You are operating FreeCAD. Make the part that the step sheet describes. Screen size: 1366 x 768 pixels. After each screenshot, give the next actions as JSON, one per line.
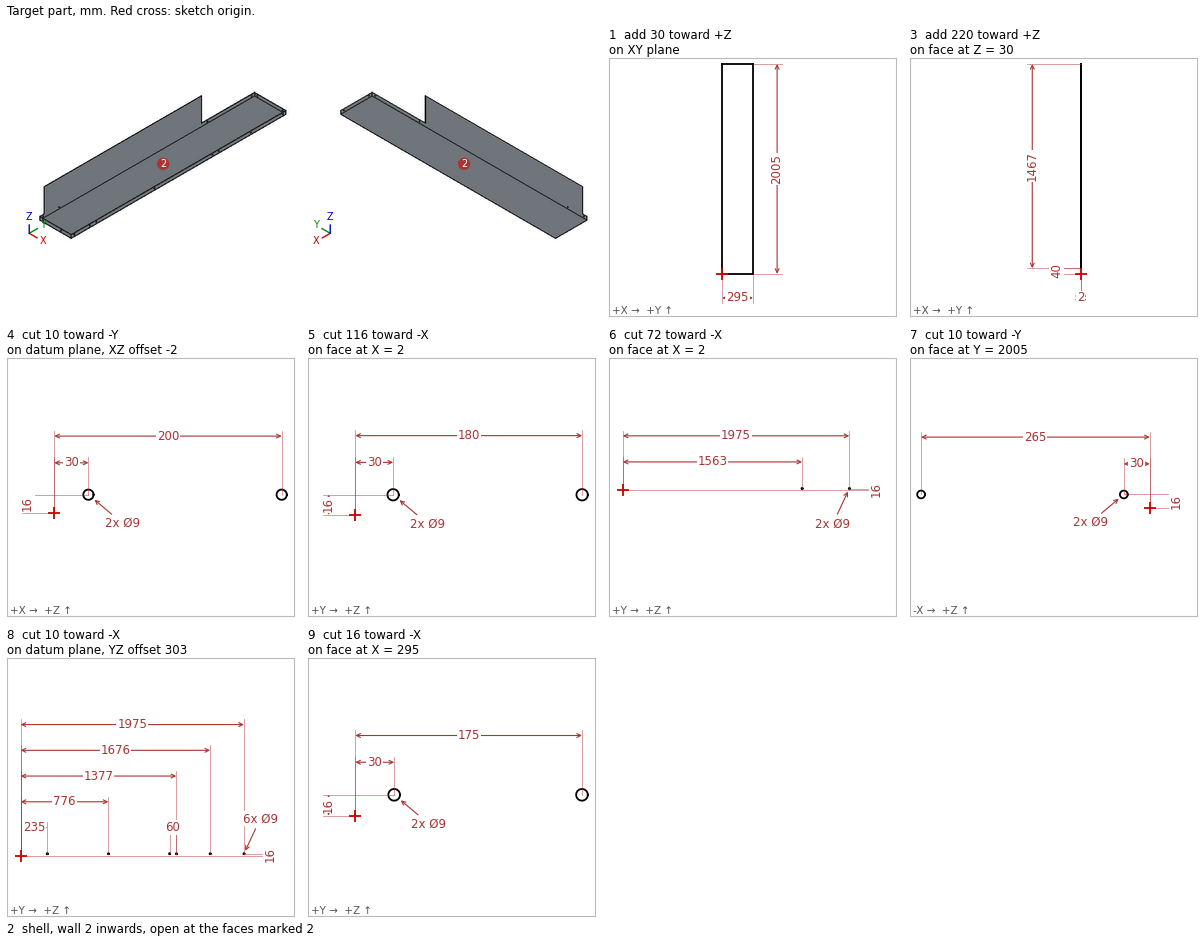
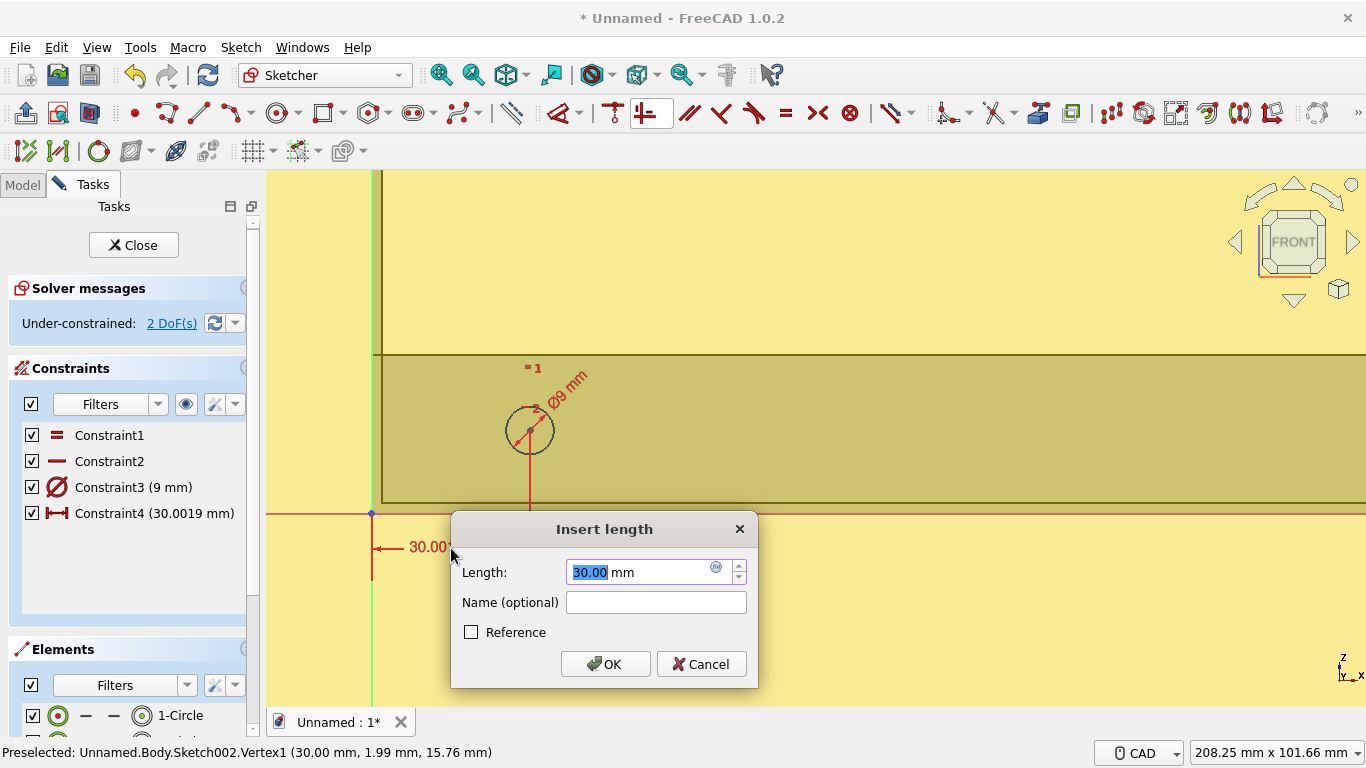
{"action": "type", "text": "30"}
{"action": "key", "text": "Return"}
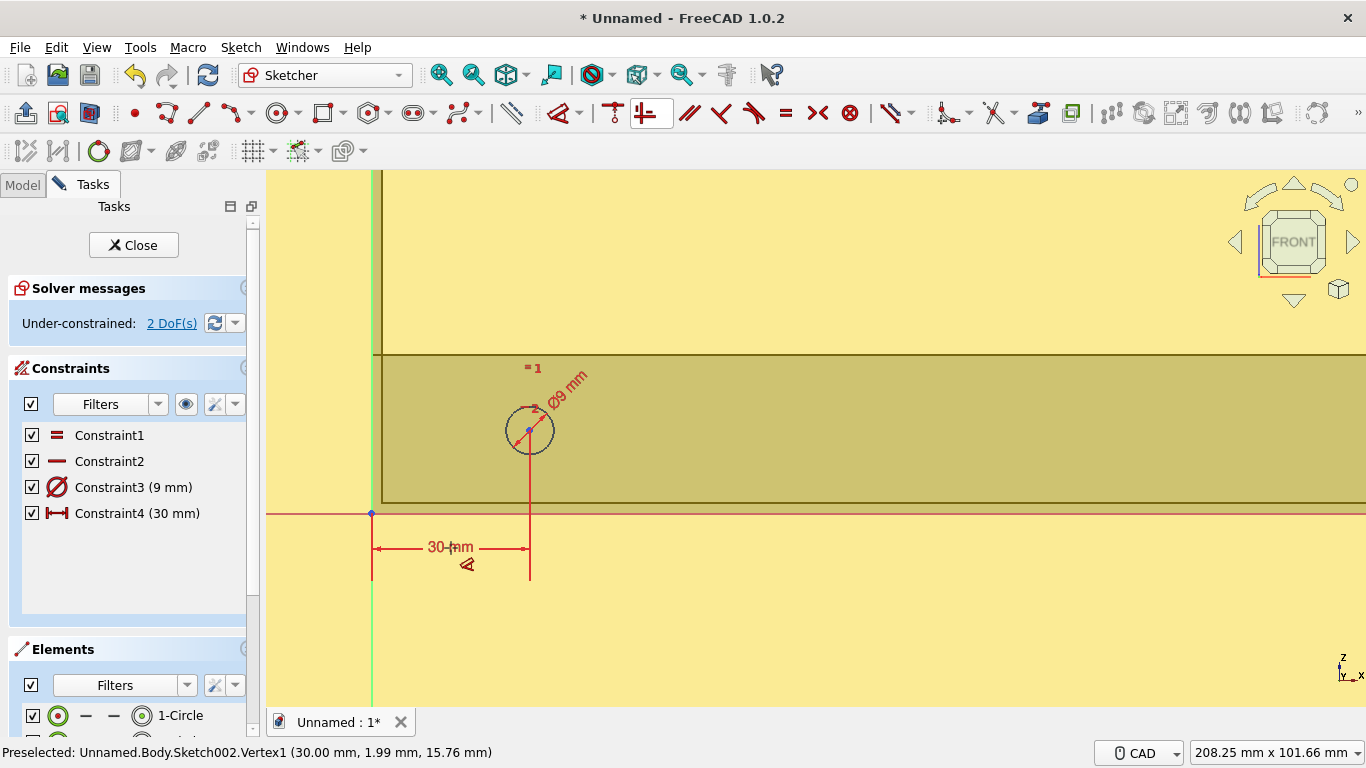
{"action": "left_click", "coordinate": [530, 430]}
{"action": "left_click", "coordinate": [338, 472]}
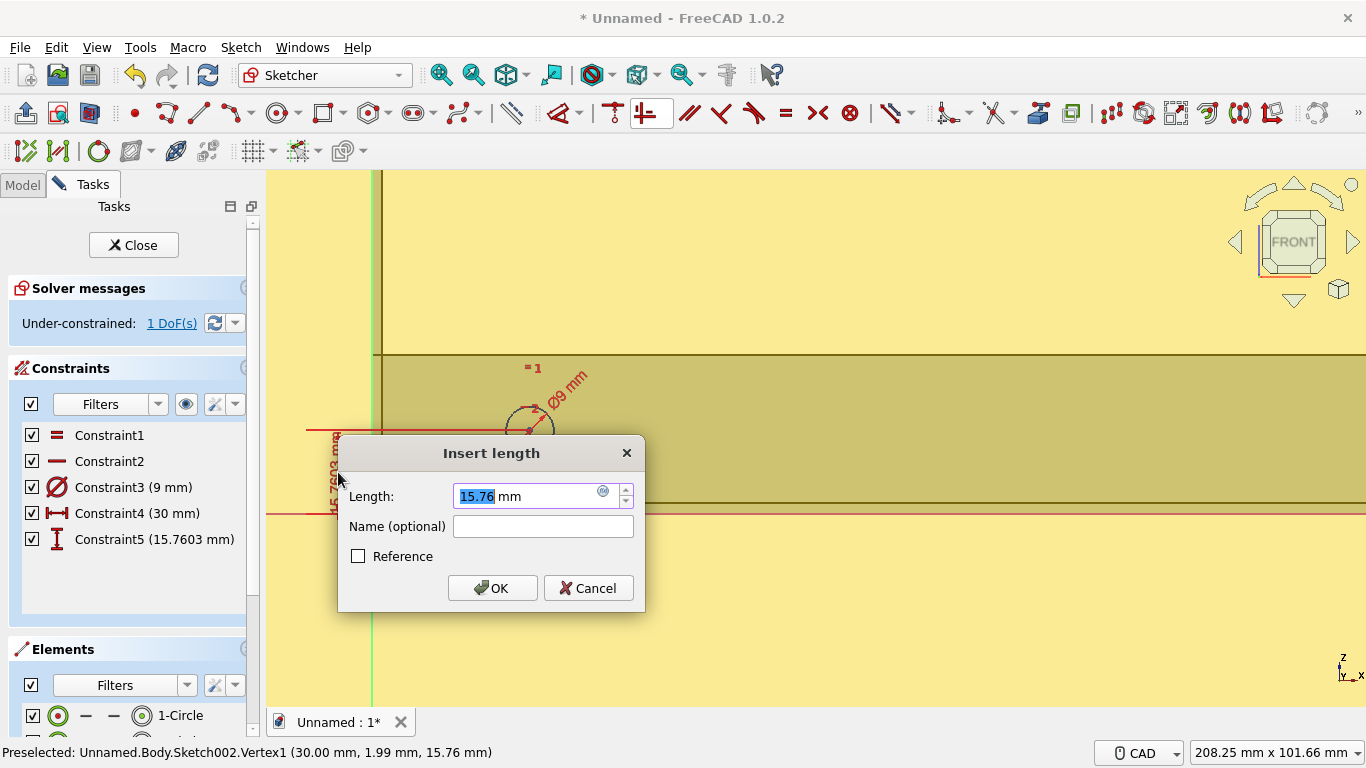
{"action": "type", "text": "16"}
{"action": "key", "text": "Return"}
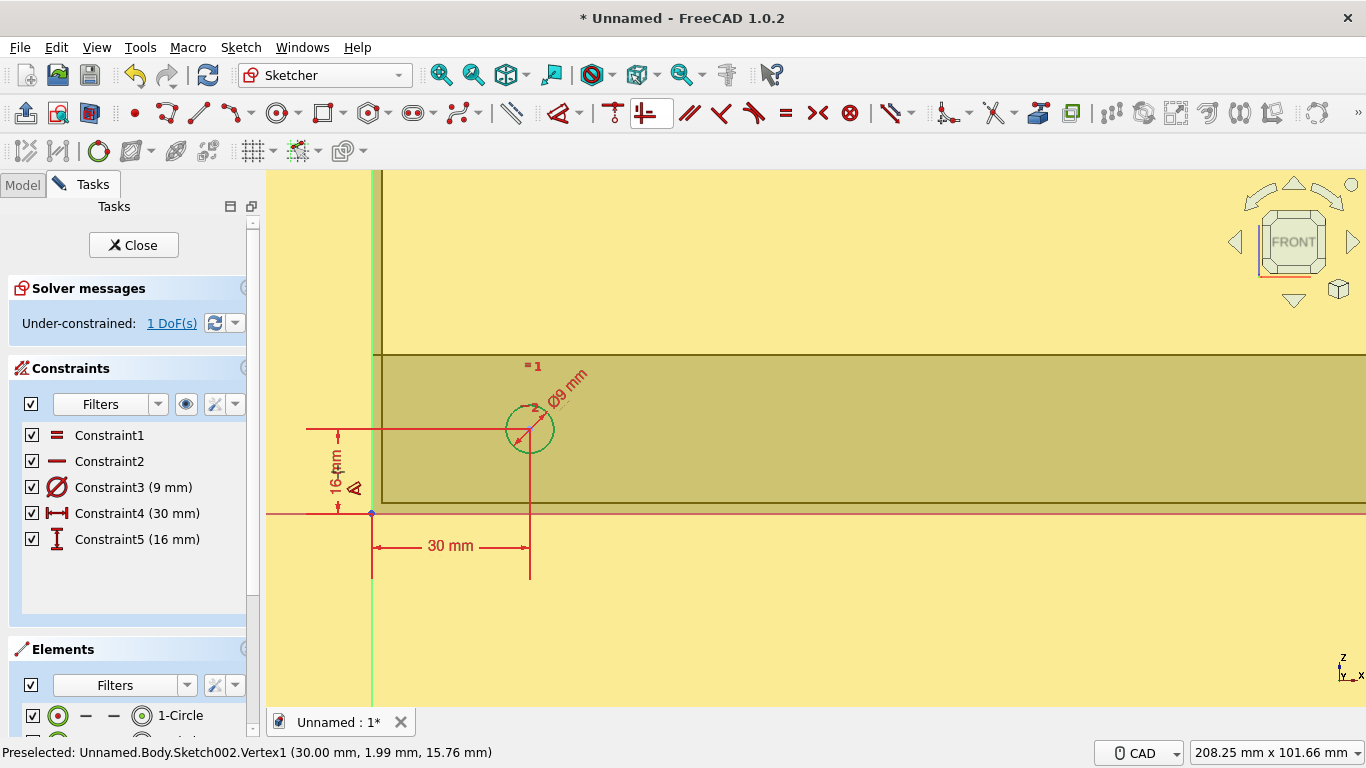
{"action": "scroll", "coordinate": [548, 413], "scroll_direction": "down", "scroll_amount": 3}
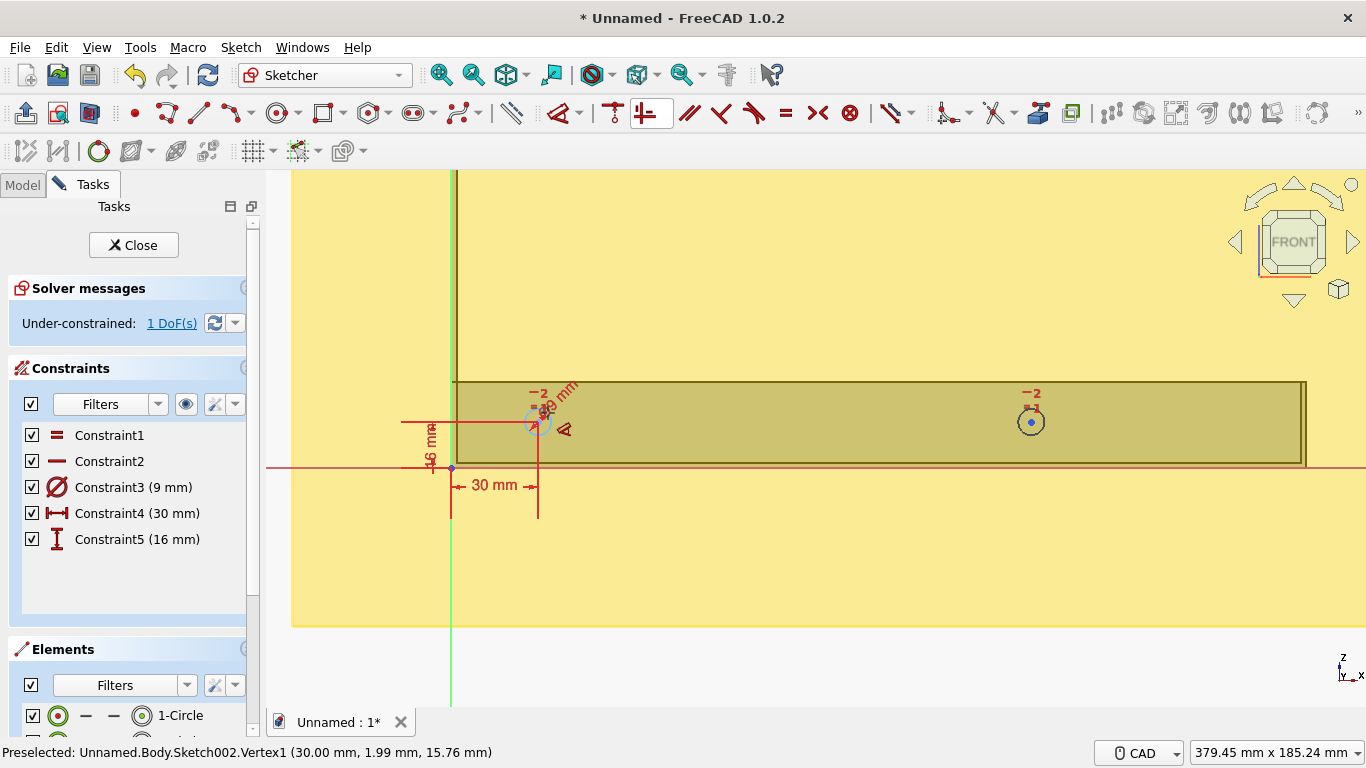
{"action": "left_click", "coordinate": [1031, 422]}
{"action": "left_click", "coordinate": [741, 502]}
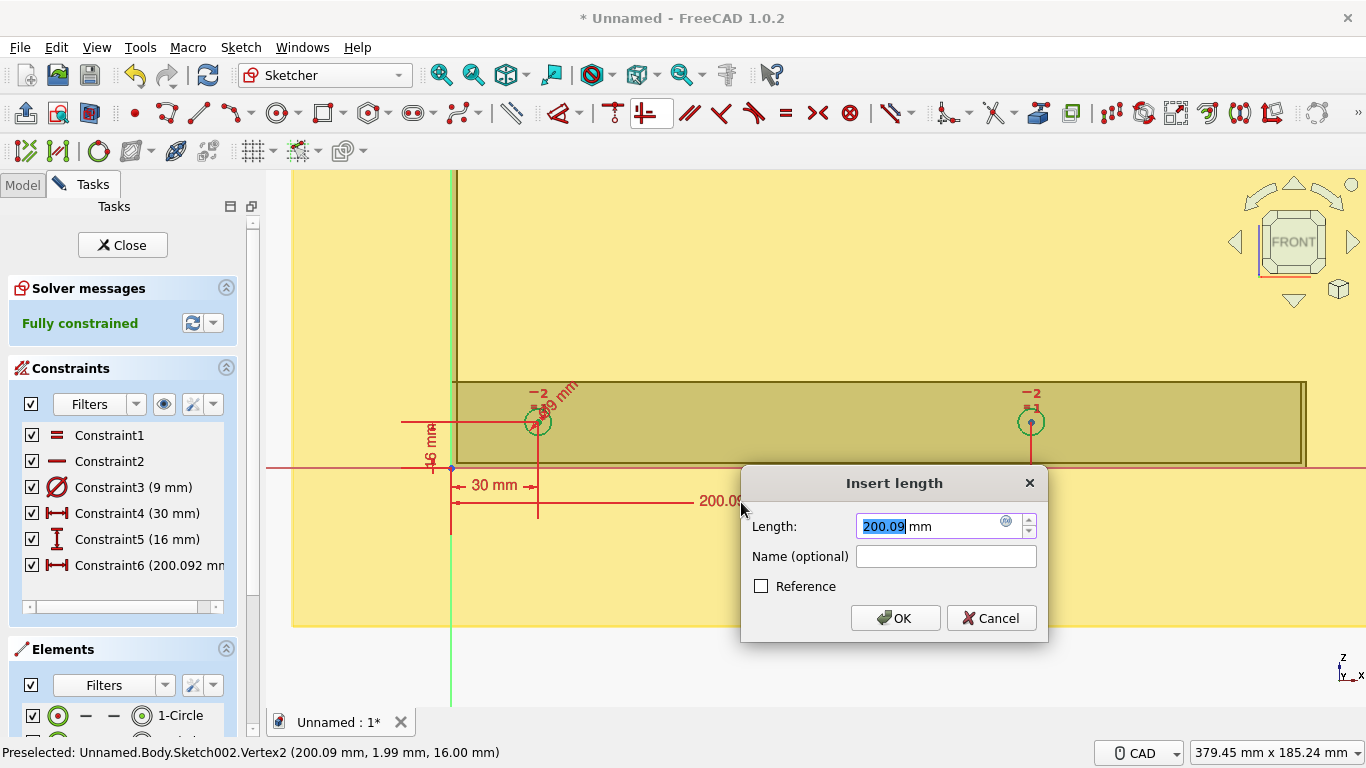
{"action": "type", "text": "200"}
{"action": "key", "text": "Return"}
{"action": "key", "text": "Escape"}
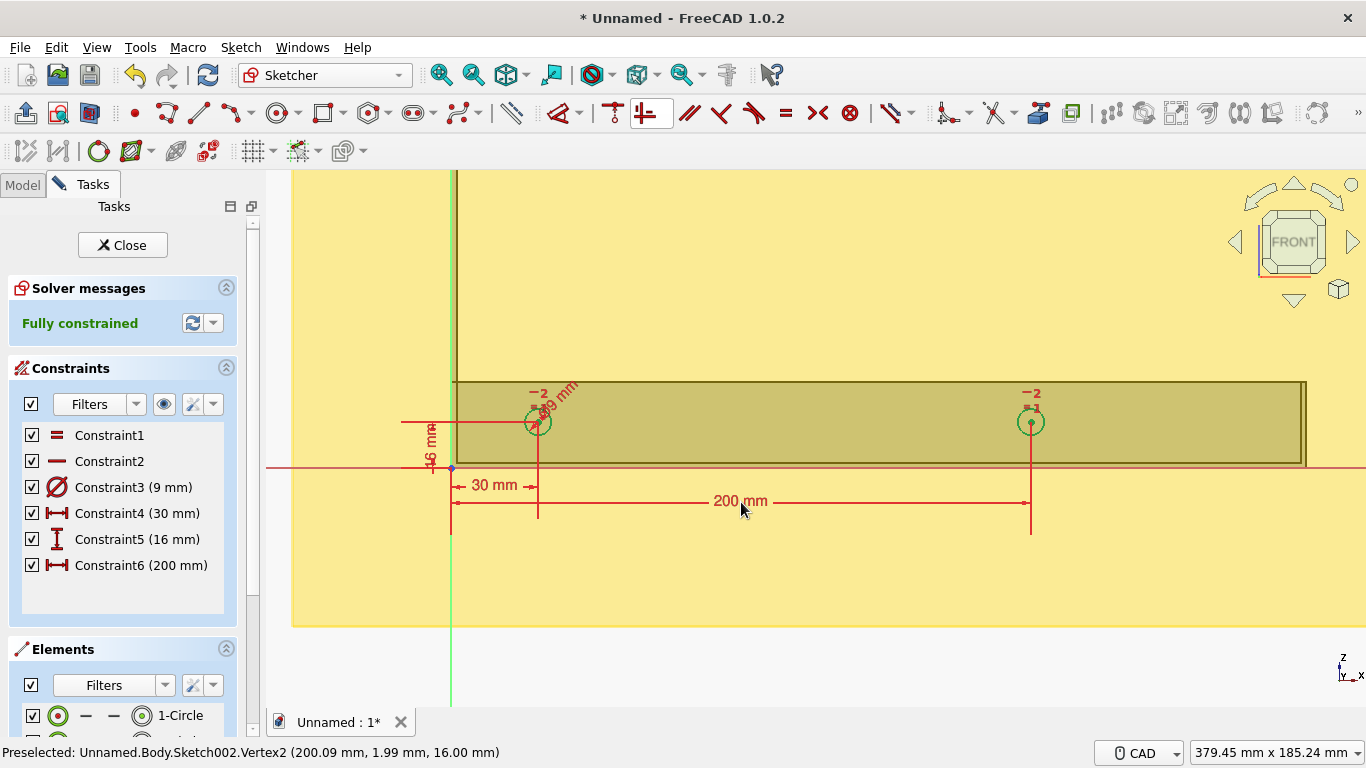
{"action": "left_click", "coordinate": [123, 245]}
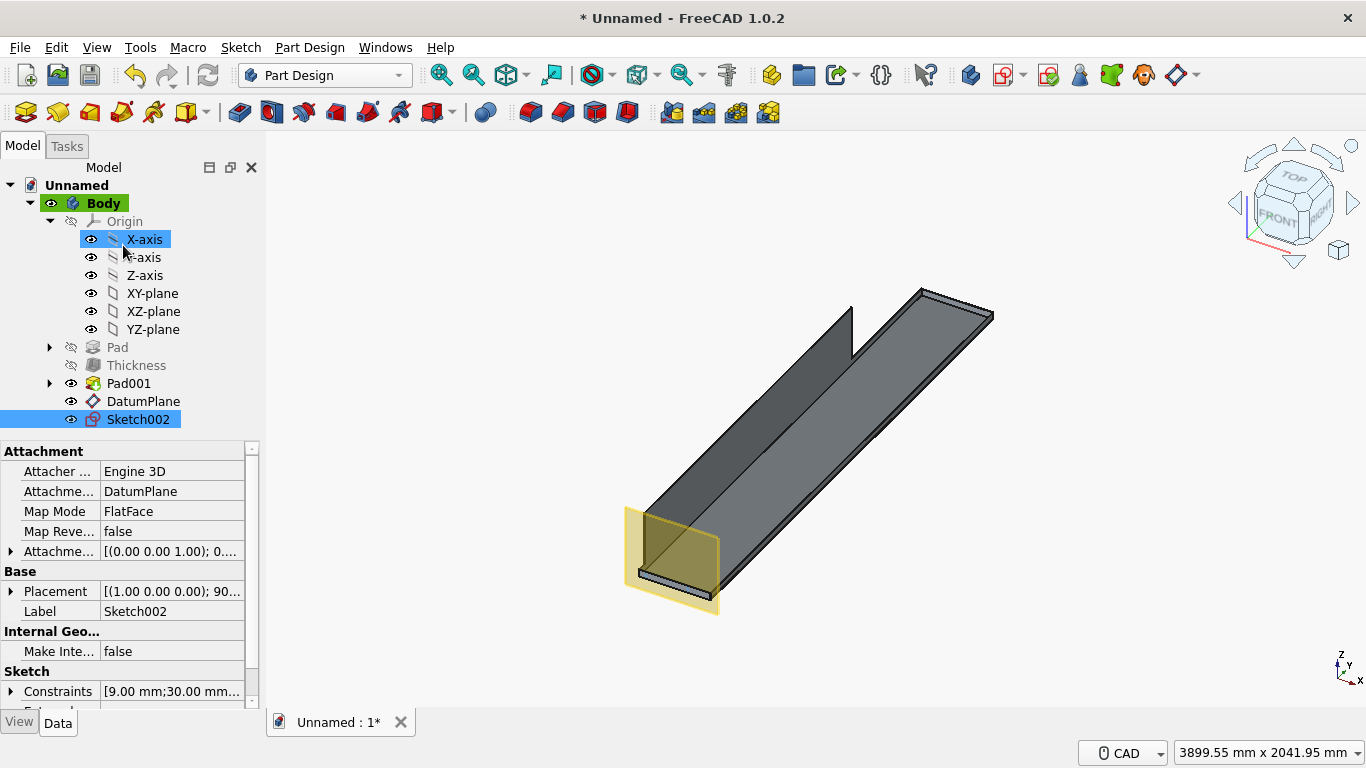
{"action": "left_click", "coordinate": [240, 112]}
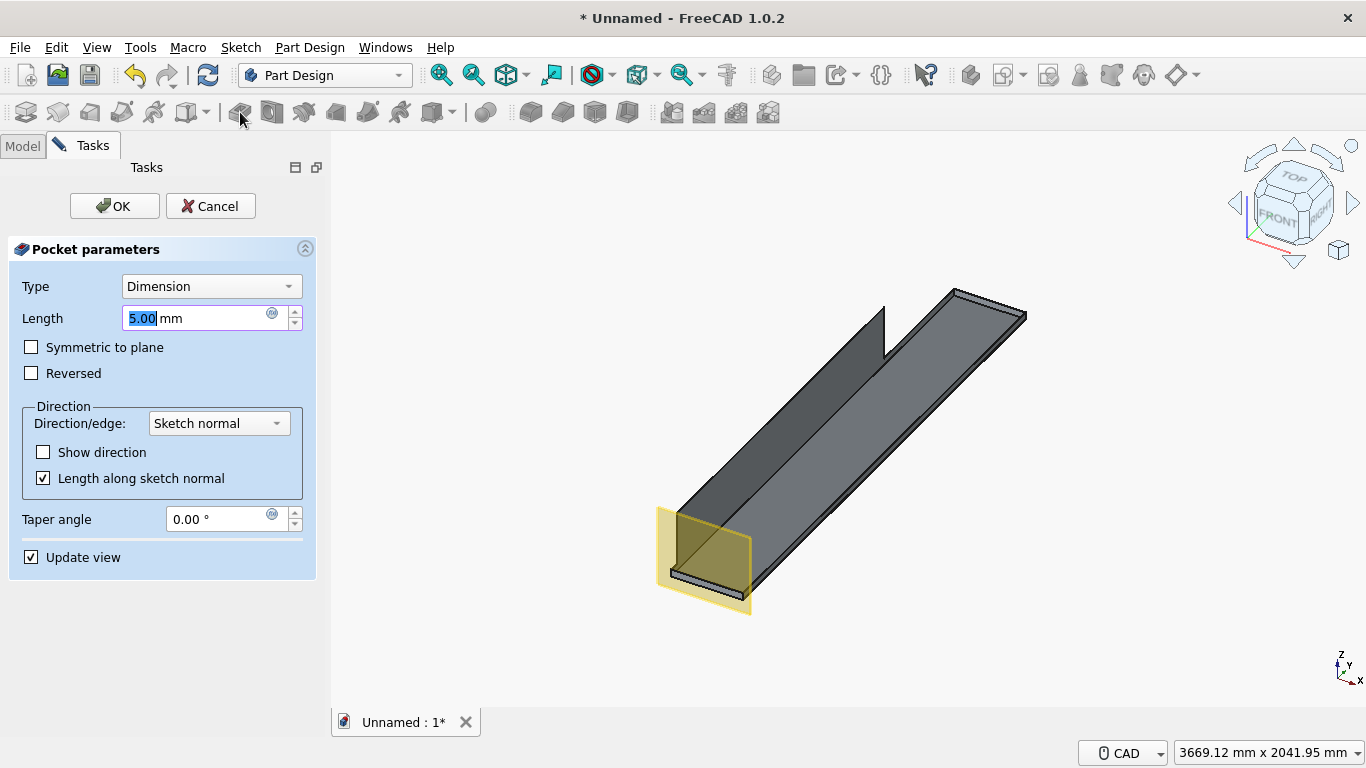
{"action": "type", "text": "10"}
{"action": "key", "text": "Tab"}